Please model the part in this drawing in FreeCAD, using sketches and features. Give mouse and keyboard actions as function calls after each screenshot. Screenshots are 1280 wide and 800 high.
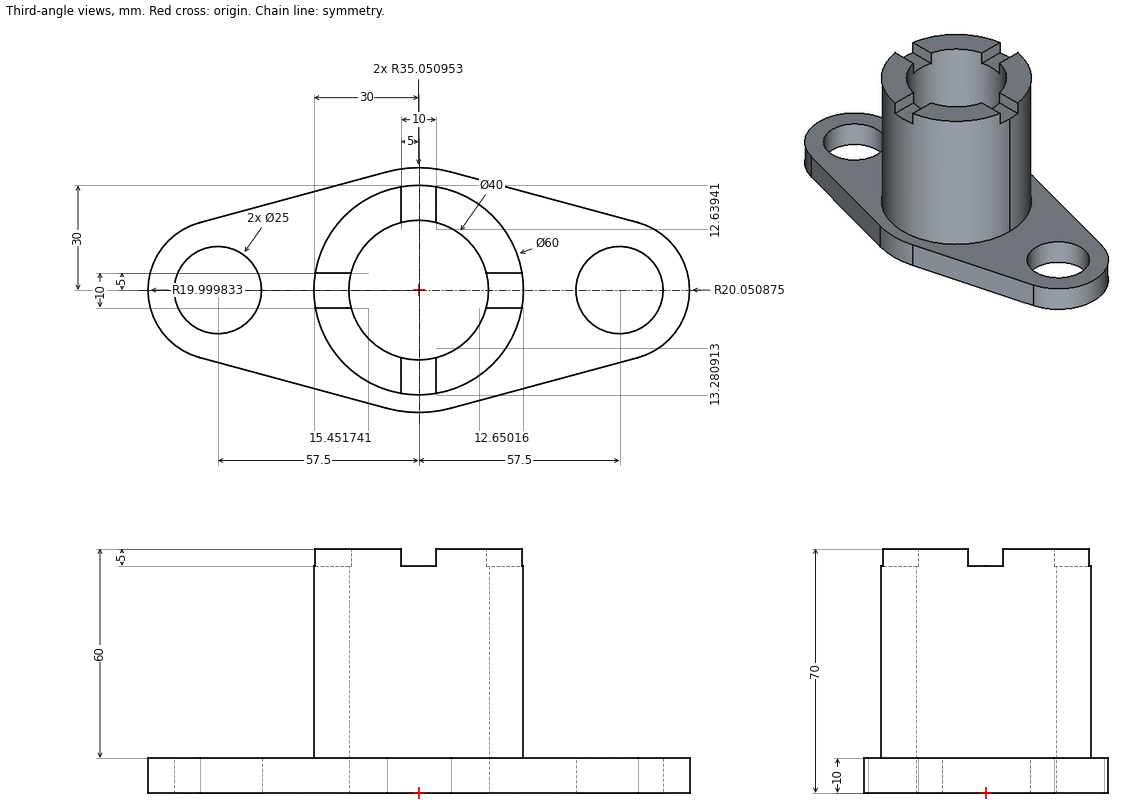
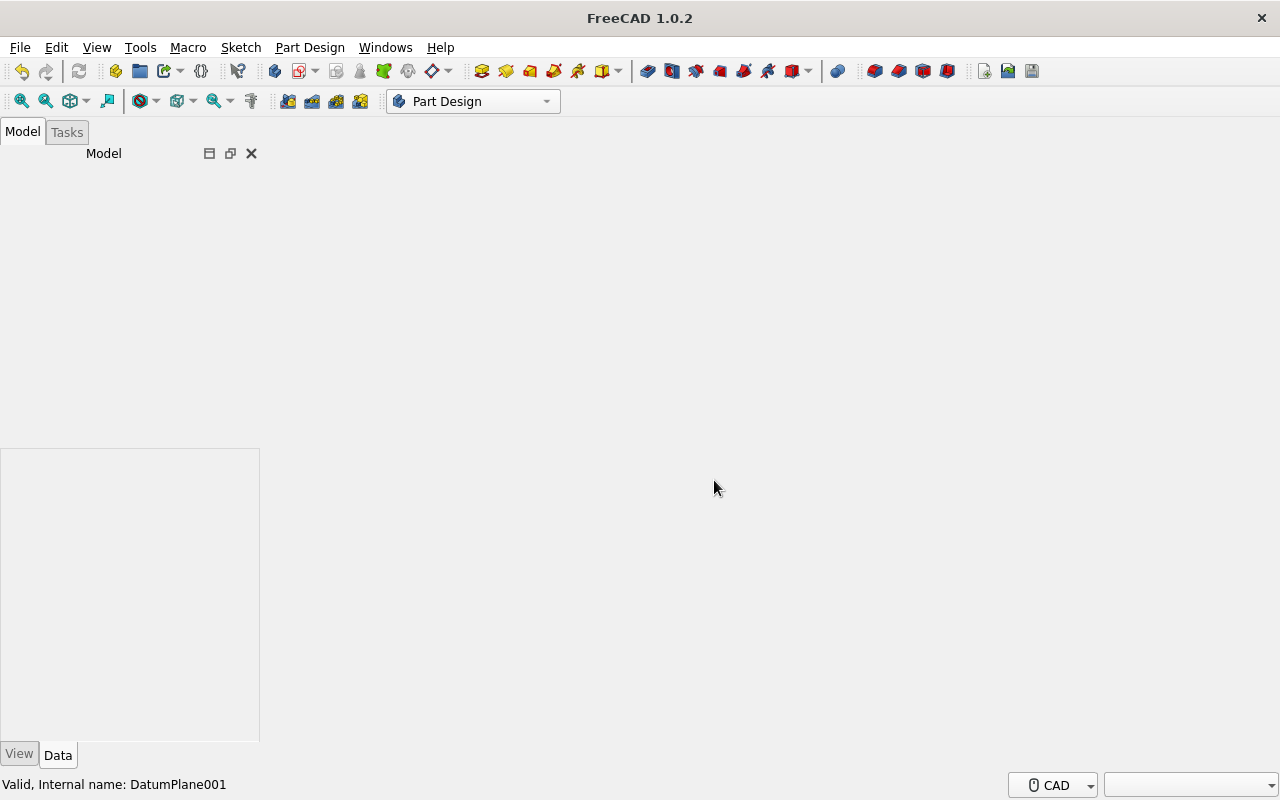
key(ctrl+n)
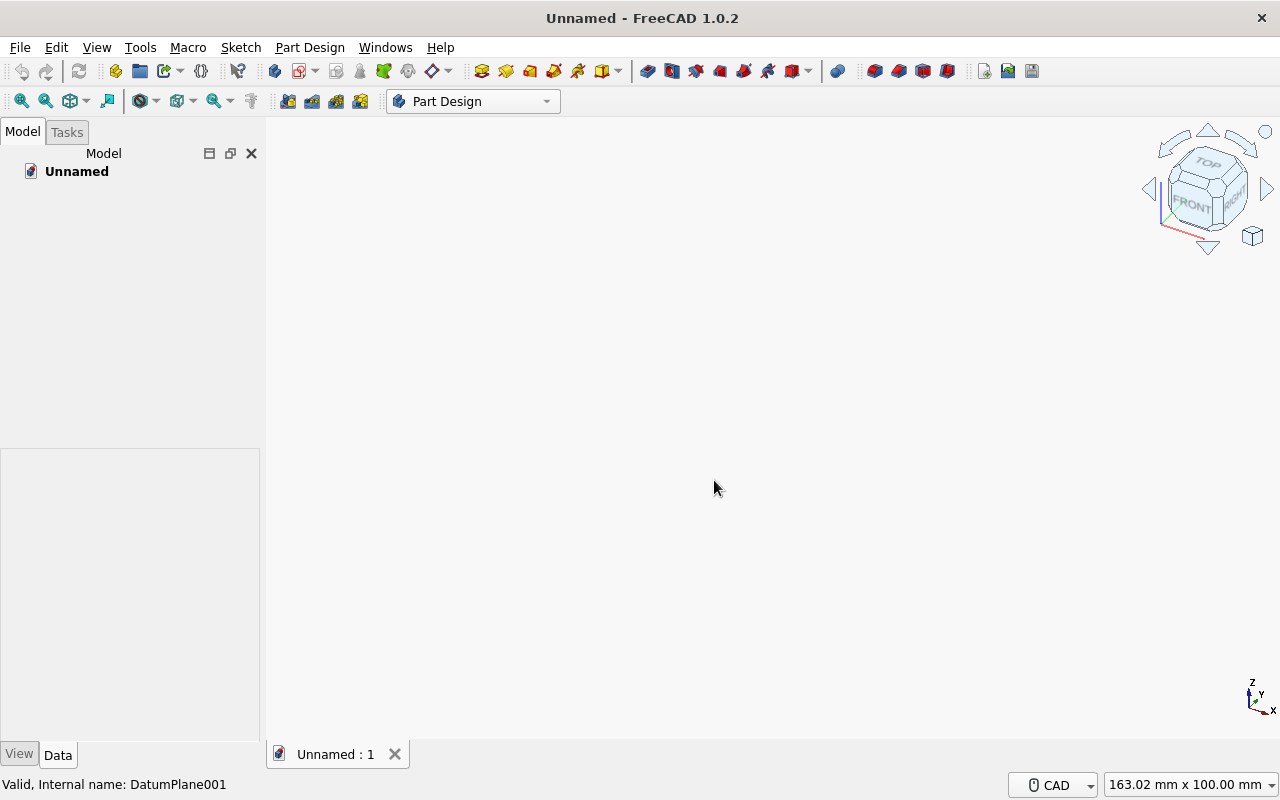
click(300, 72)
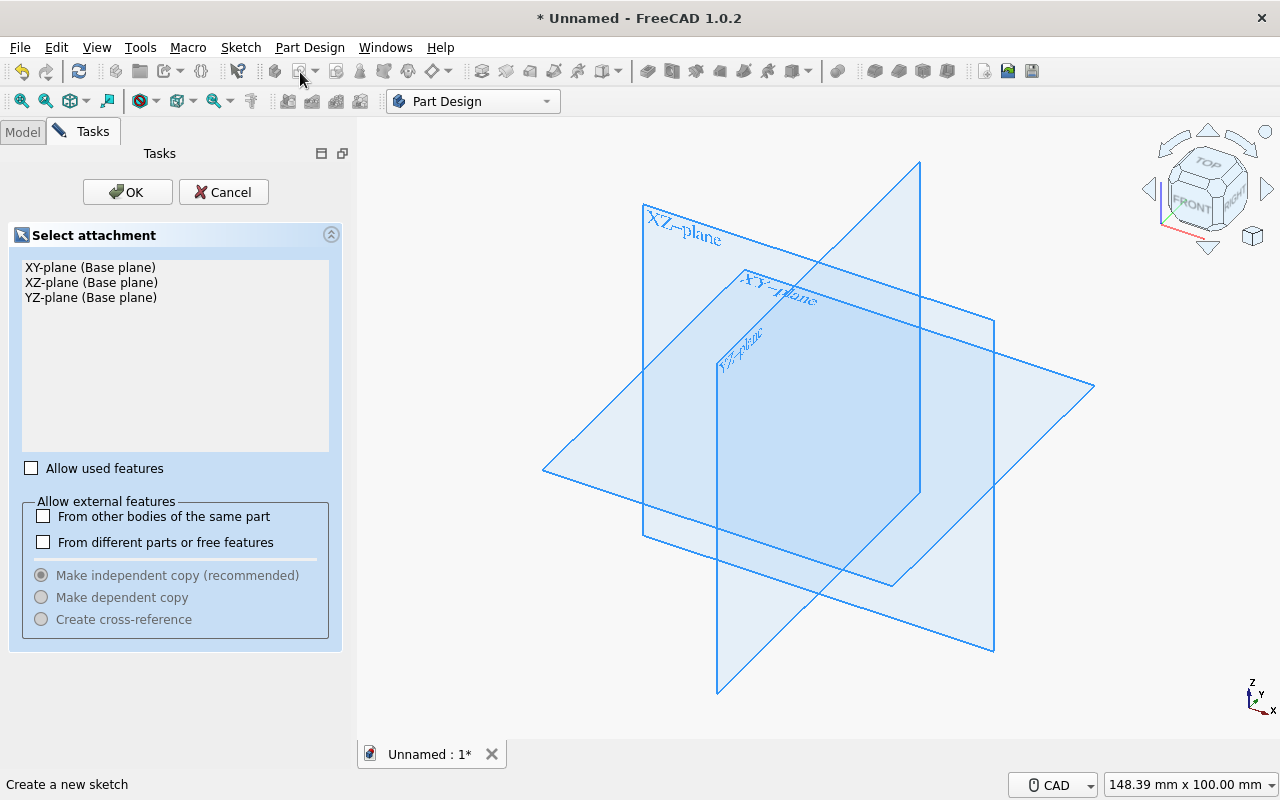
click(82, 268)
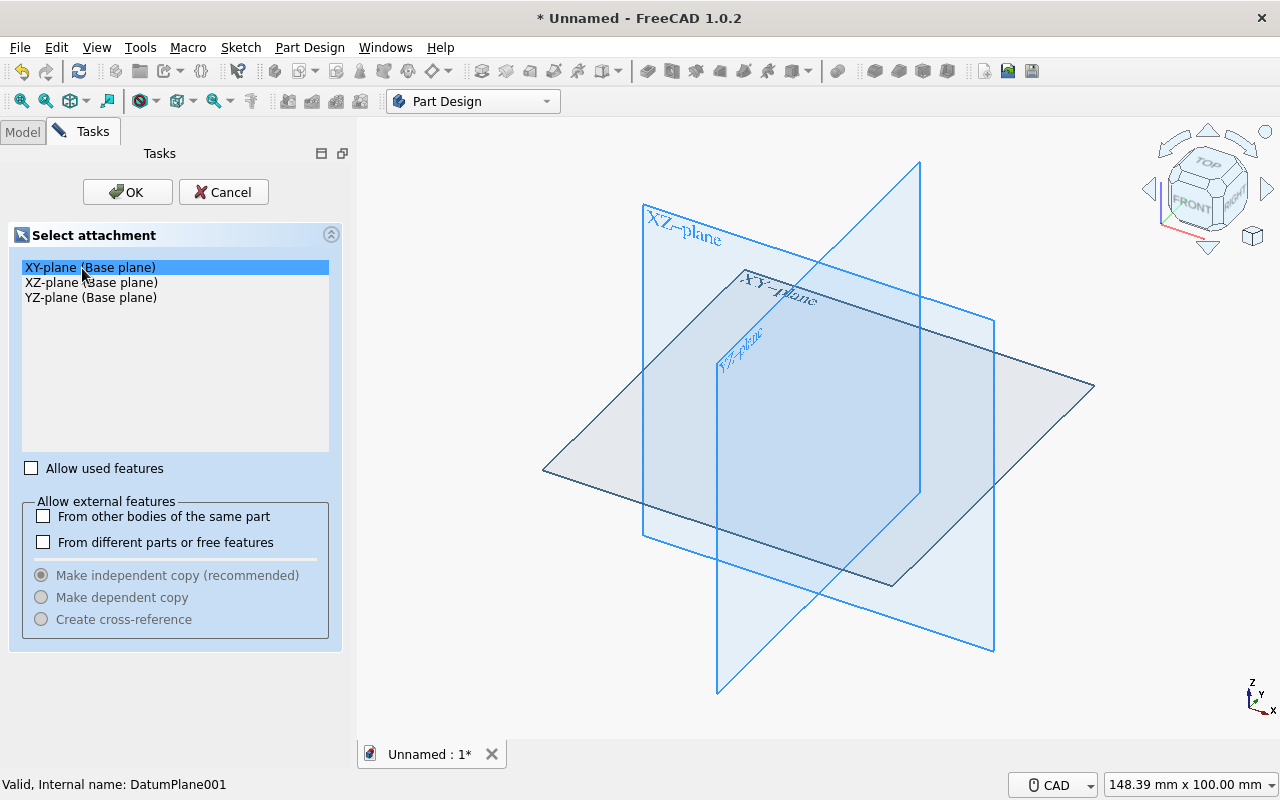
click(128, 192)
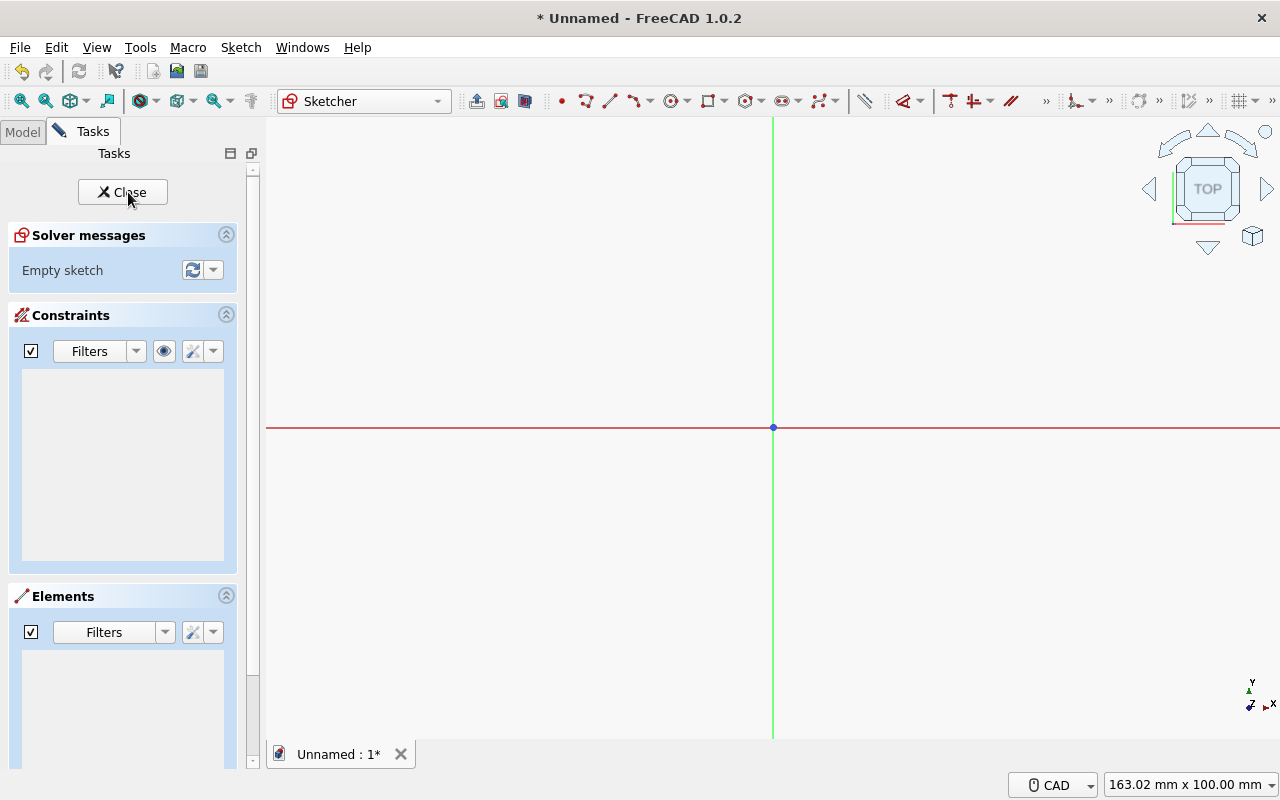
scroll(621, 428, down, 3)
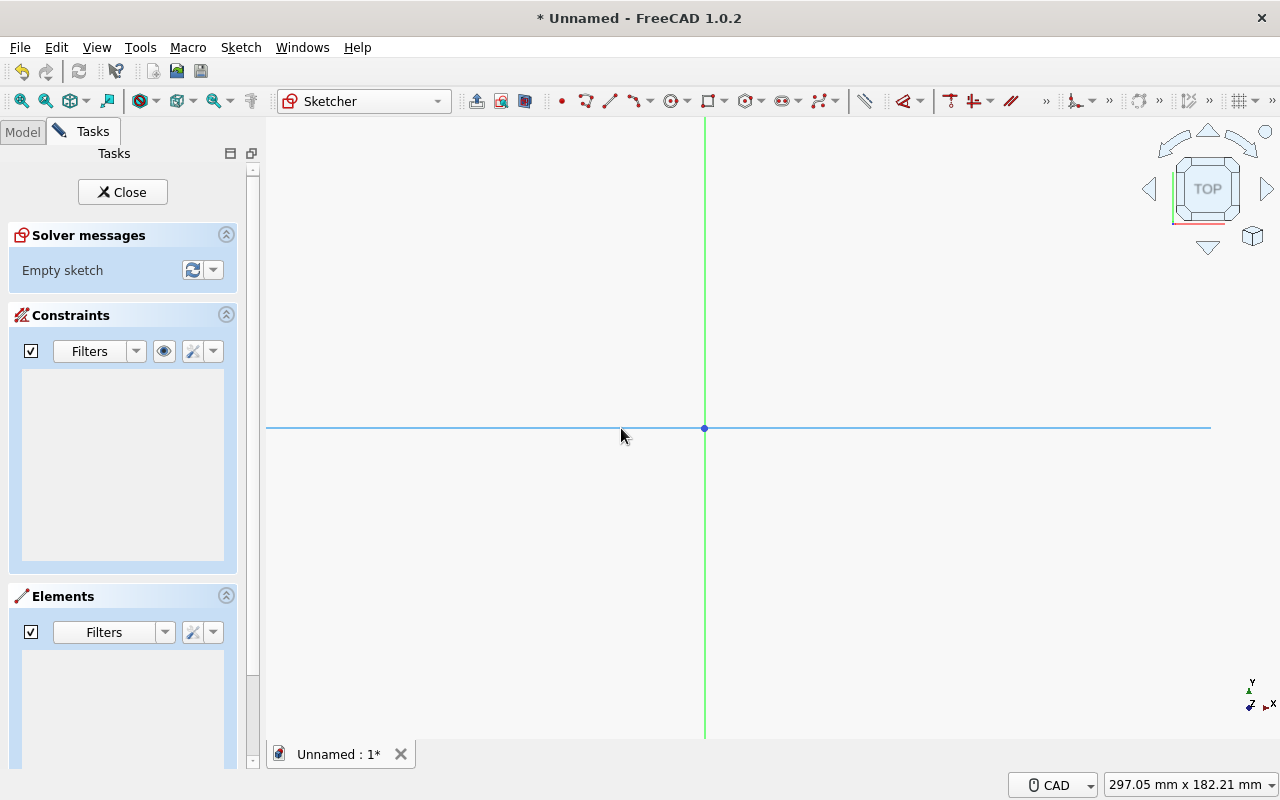
click(610, 102)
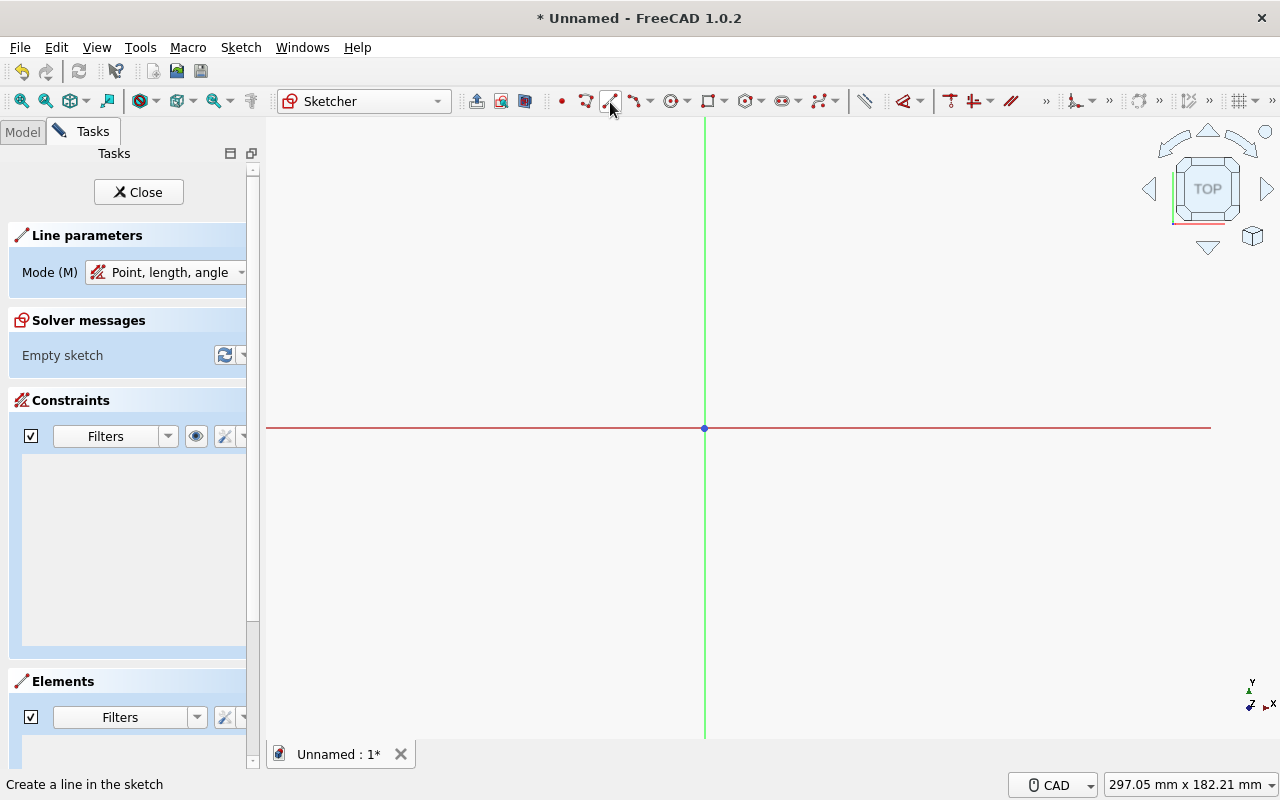
click(919, 362)
click(736, 313)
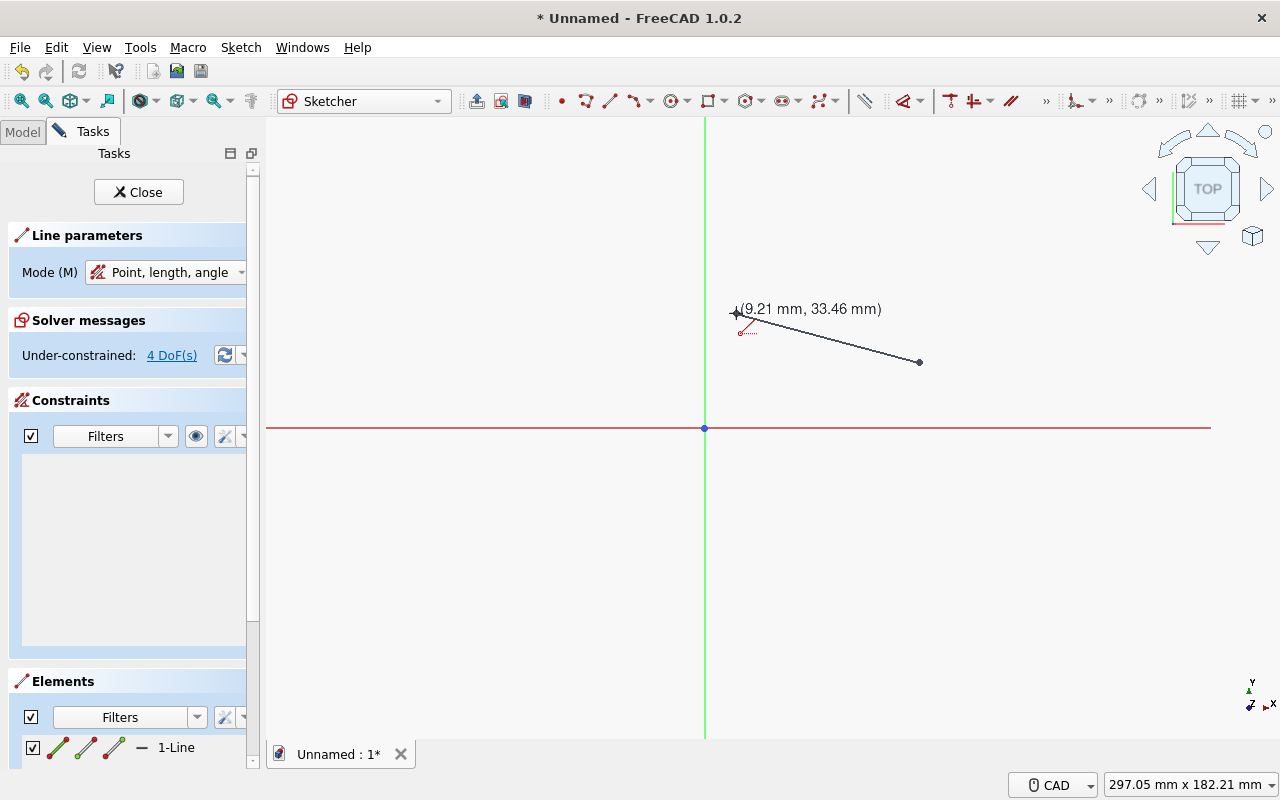
click(673, 313)
click(490, 362)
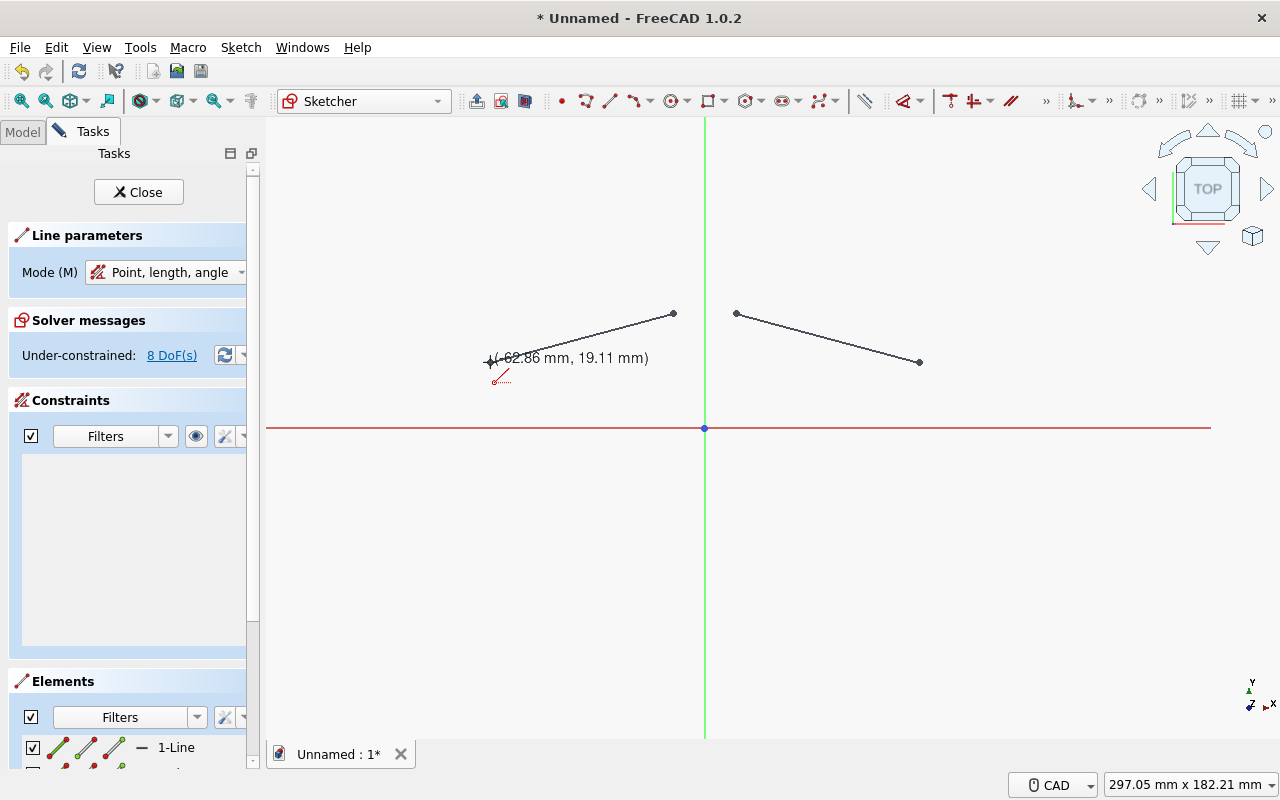
click(490, 494)
click(673, 544)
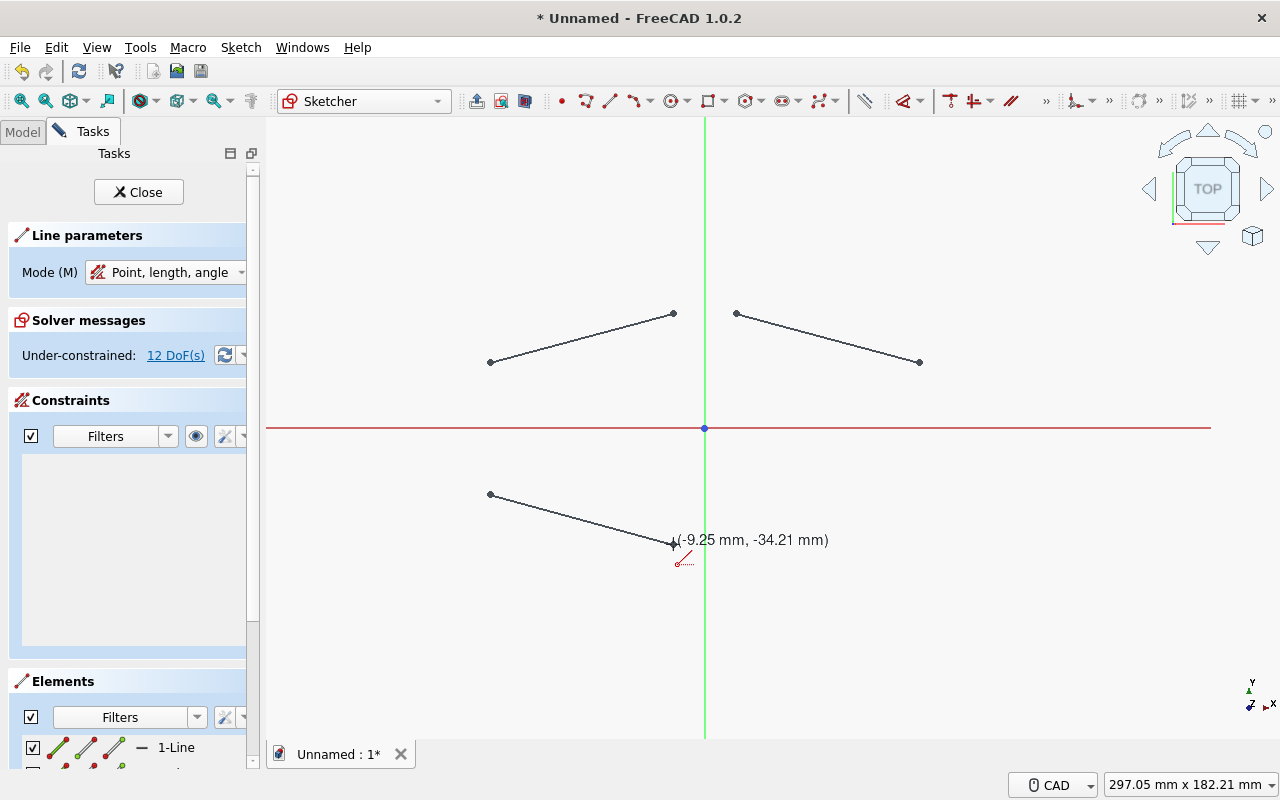
click(736, 544)
click(919, 494)